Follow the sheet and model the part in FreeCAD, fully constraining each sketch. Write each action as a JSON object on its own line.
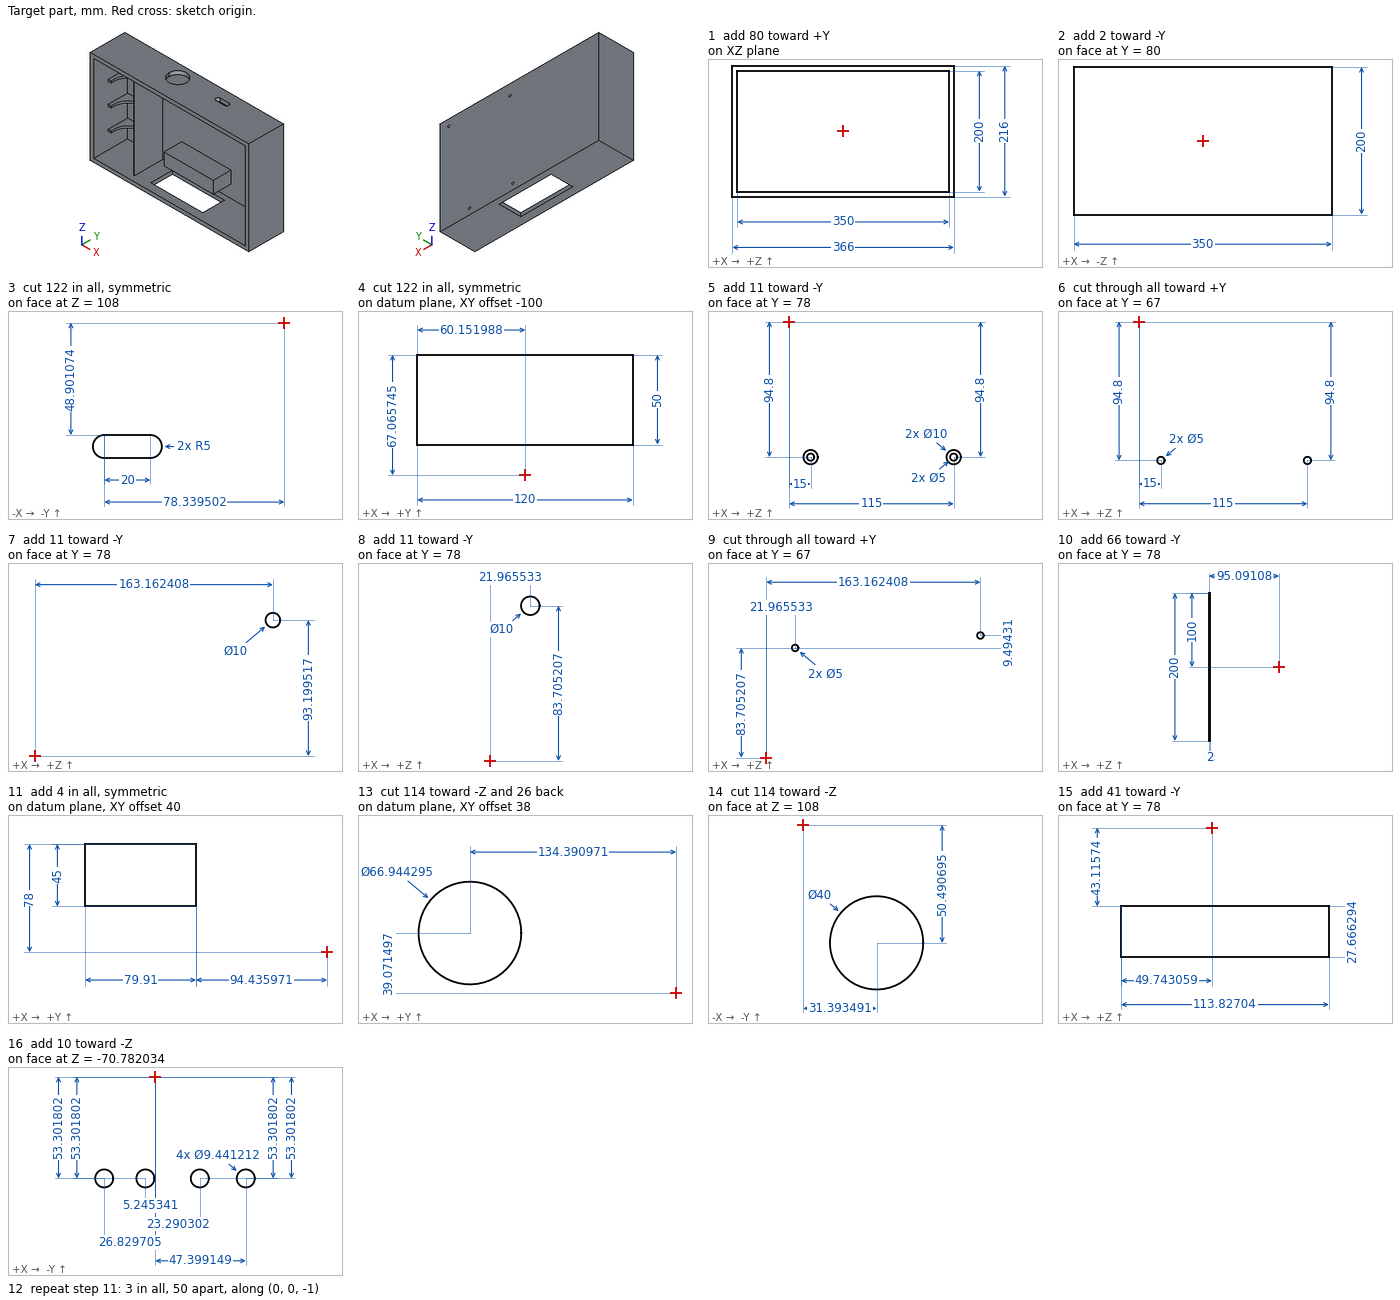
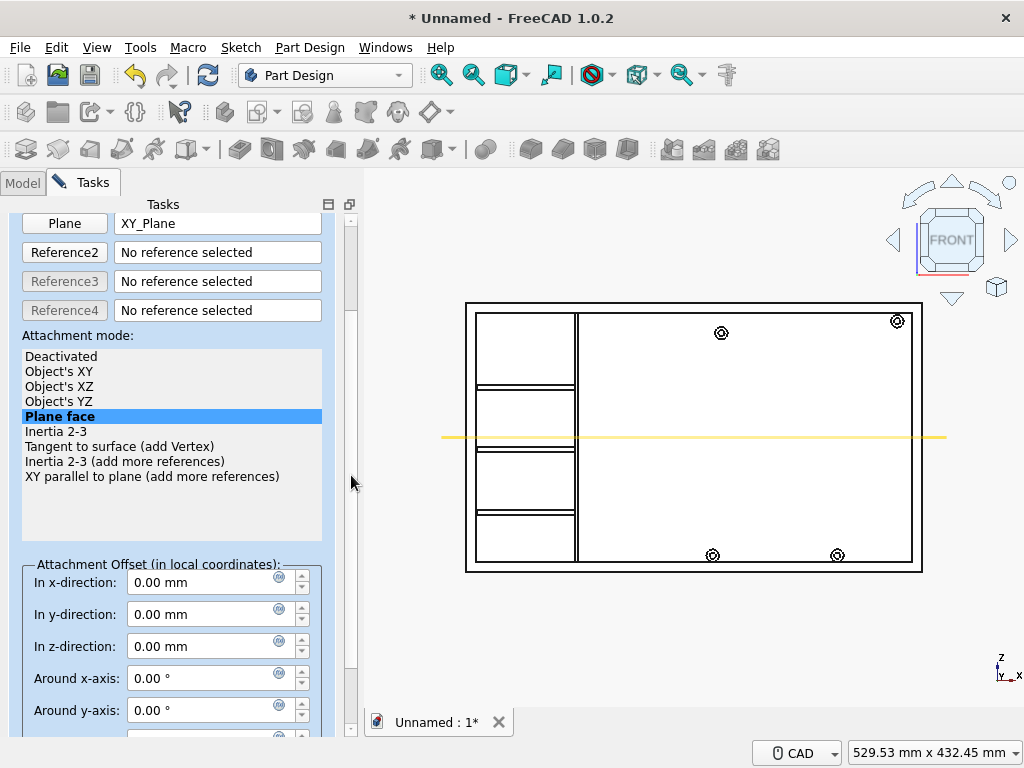
{"action": "triple_click", "coordinate": [210, 646]}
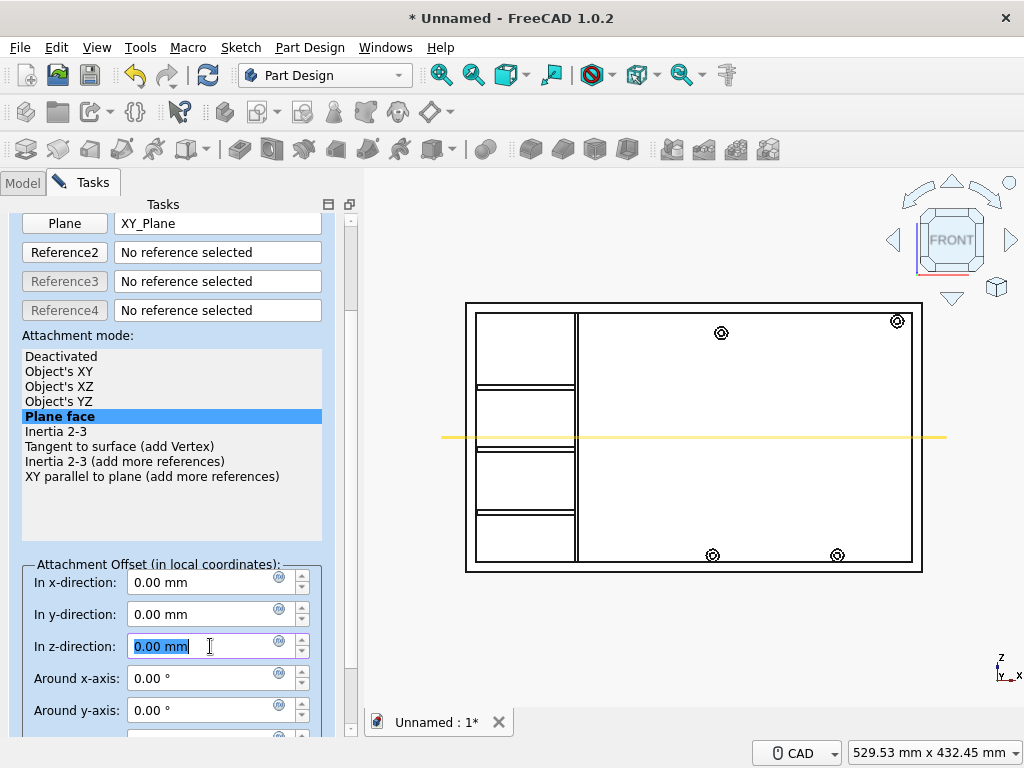
{"action": "type", "text": "38"}
{"action": "key", "text": "Tab"}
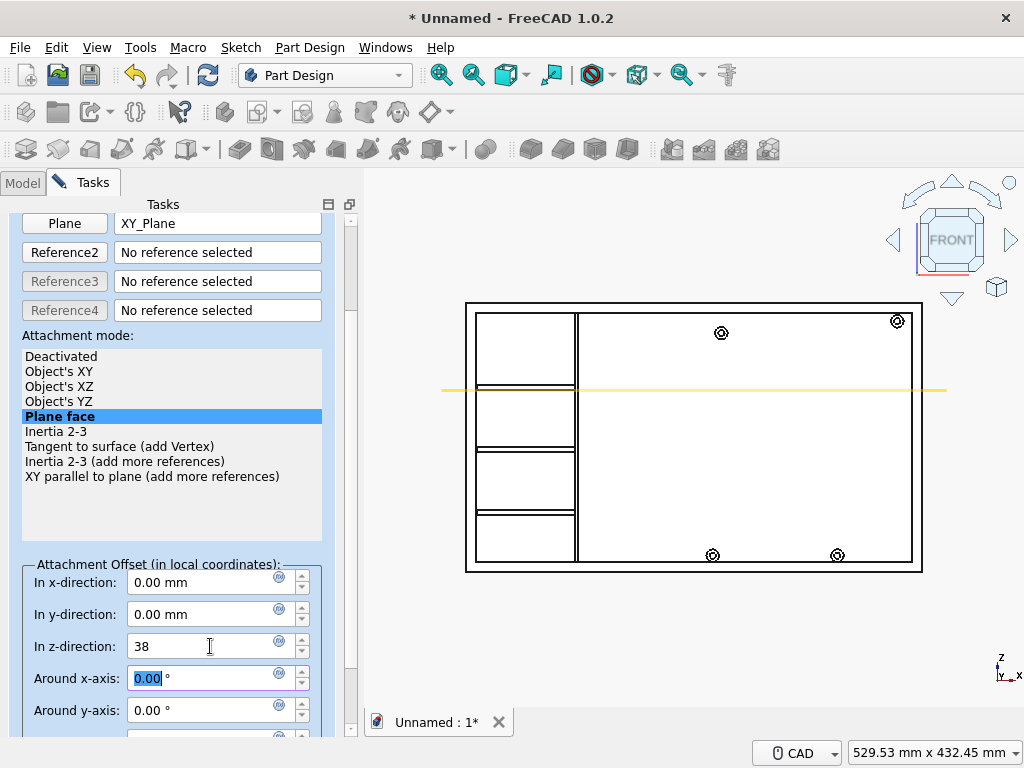
{"action": "scroll", "coordinate": [351, 475], "scroll_direction": "up", "scroll_amount": 3}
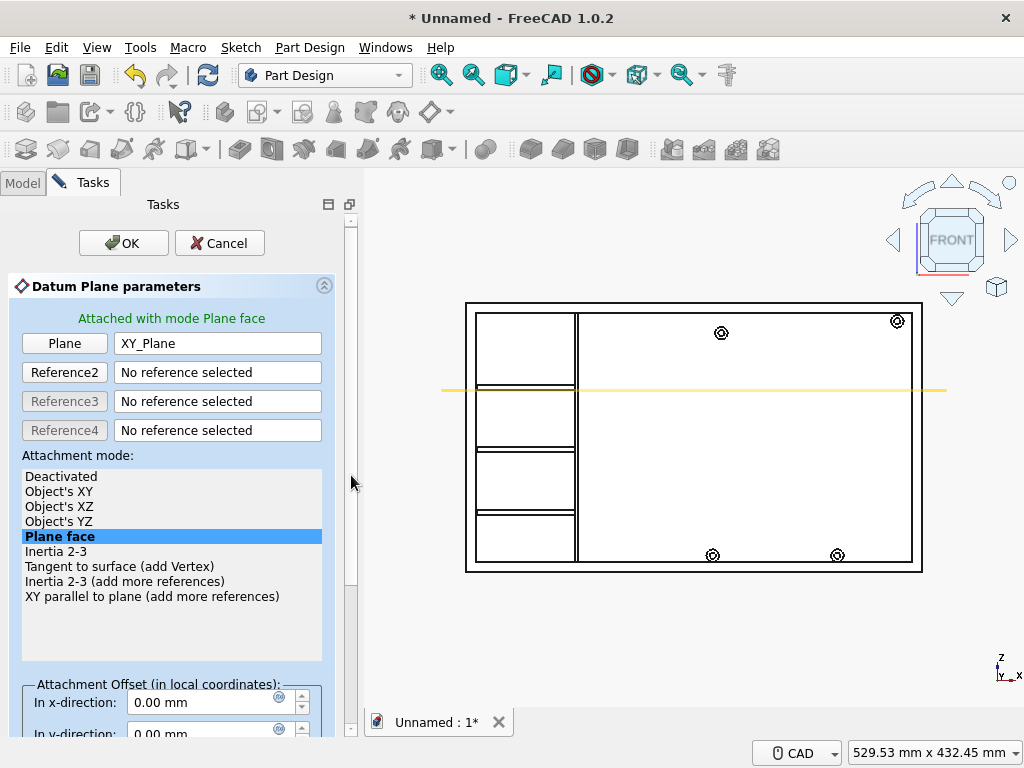
{"action": "left_click", "coordinate": [124, 243]}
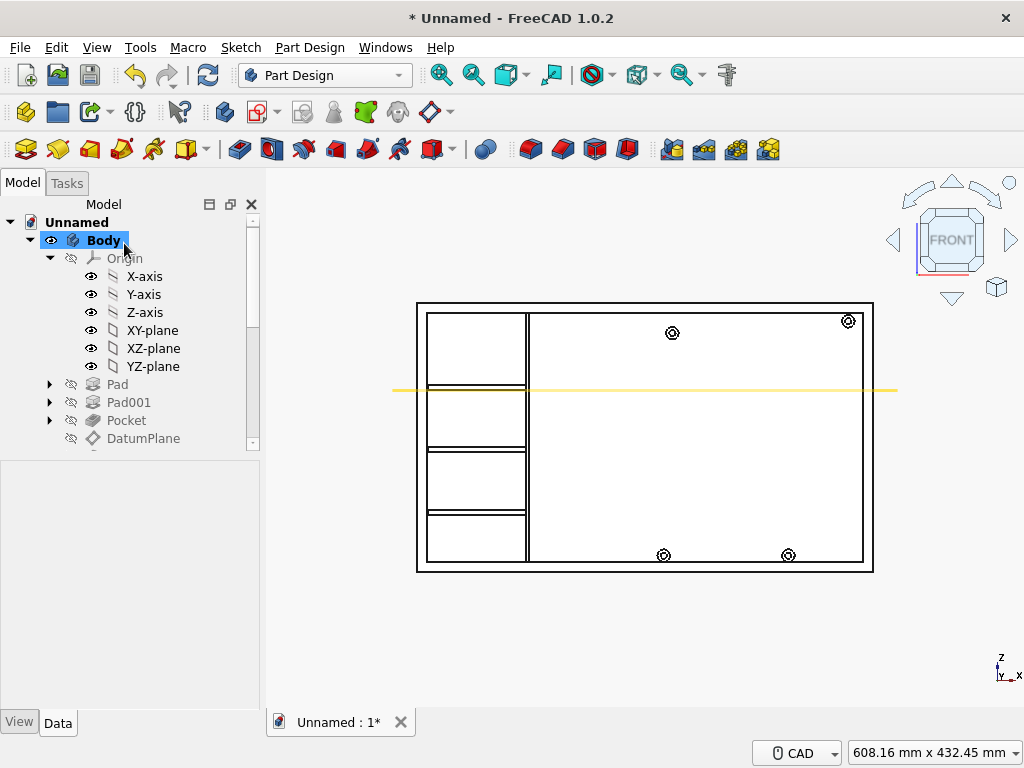
{"action": "scroll", "coordinate": [100, 326], "scroll_direction": "down", "scroll_amount": 3}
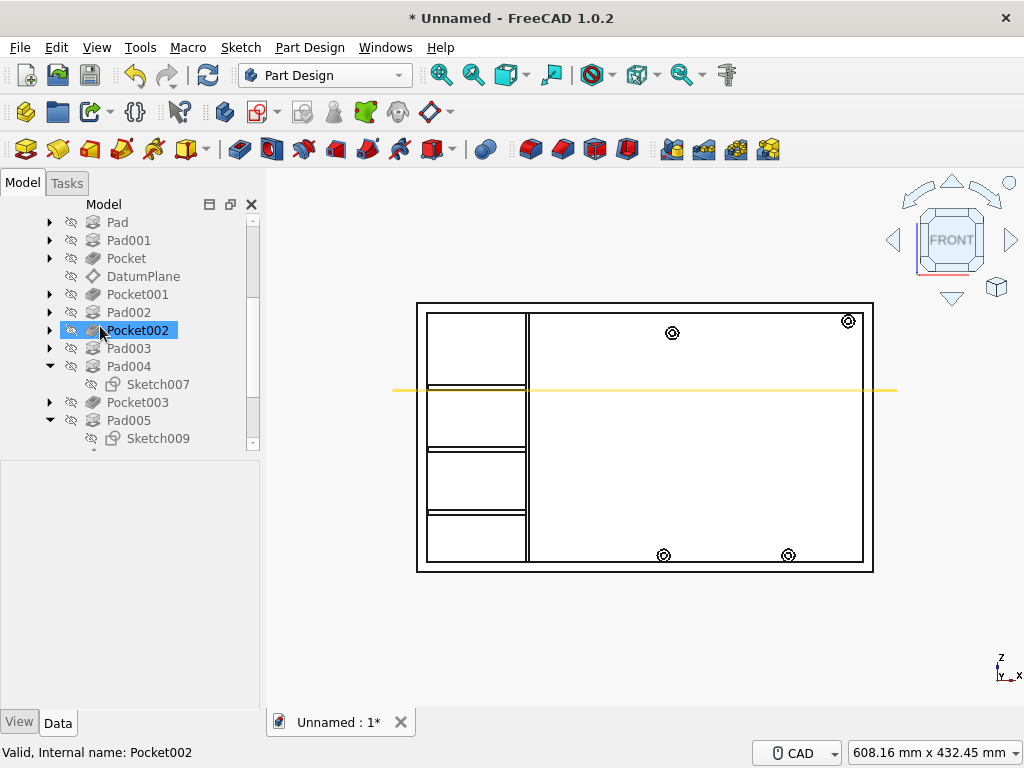
{"action": "scroll", "coordinate": [140, 326], "scroll_direction": "up", "scroll_amount": 15}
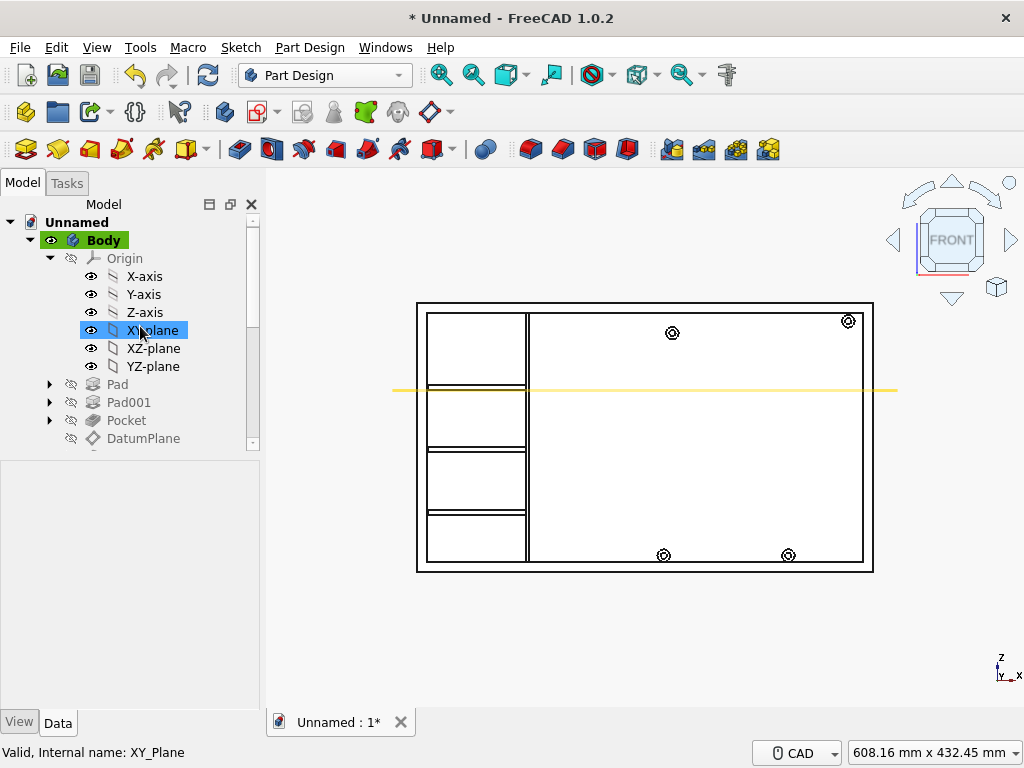
{"action": "scroll", "coordinate": [100, 326], "scroll_direction": "down", "scroll_amount": 6}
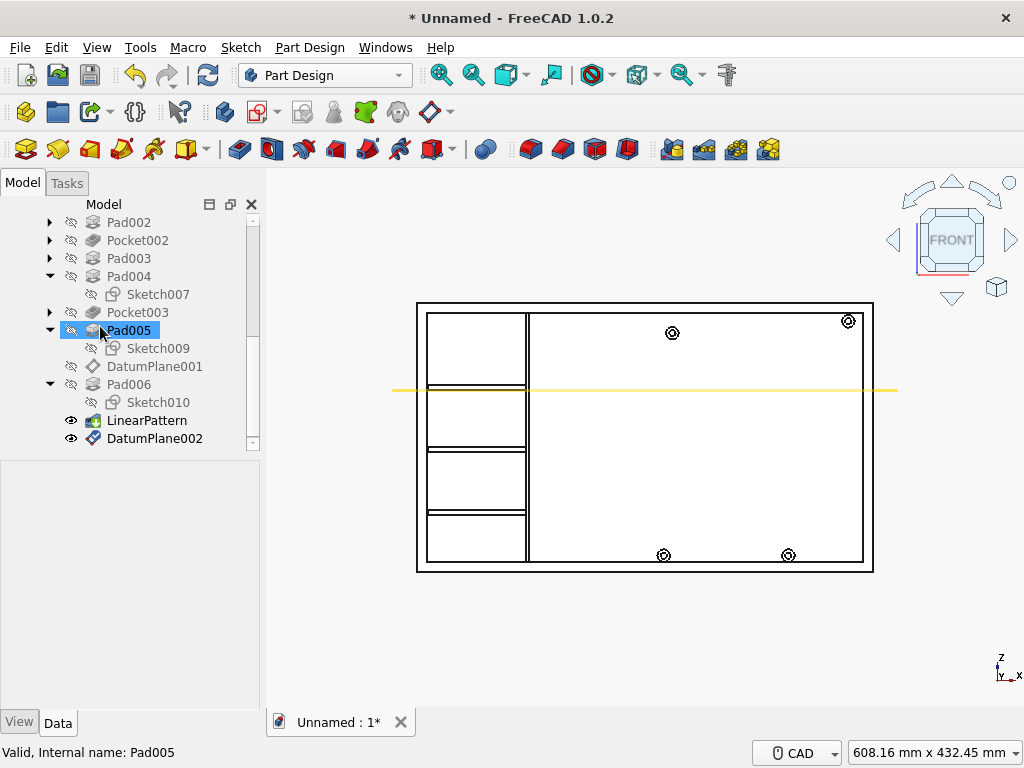
{"action": "left_click", "coordinate": [116, 438]}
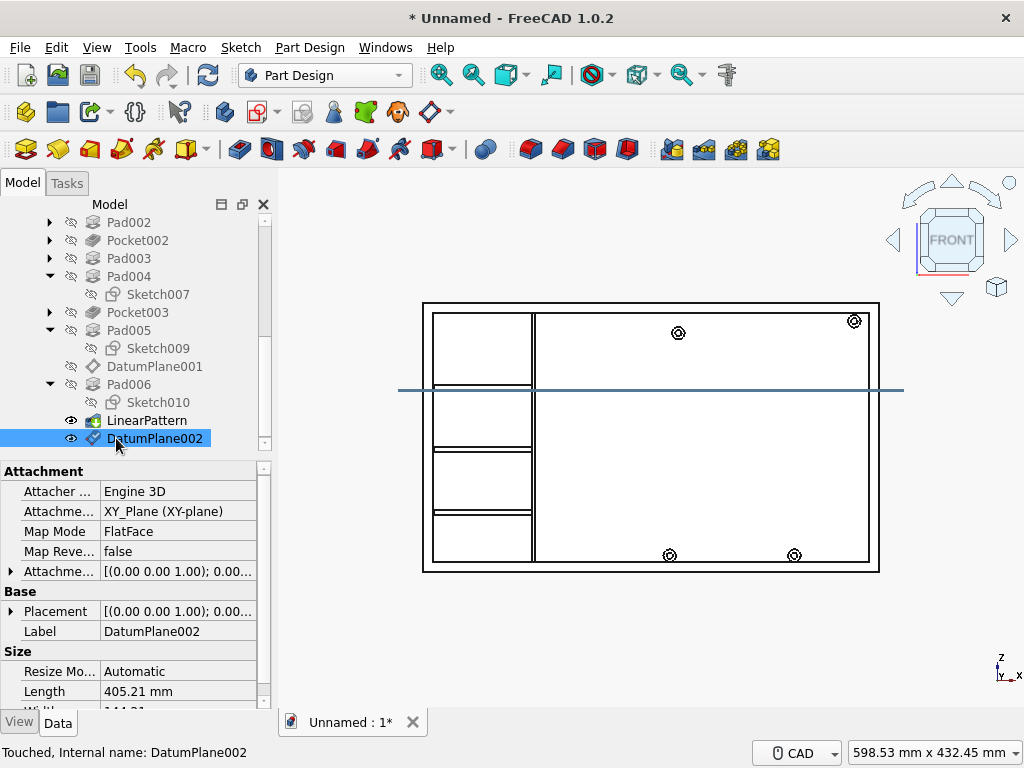
{"action": "left_click", "coordinate": [258, 112]}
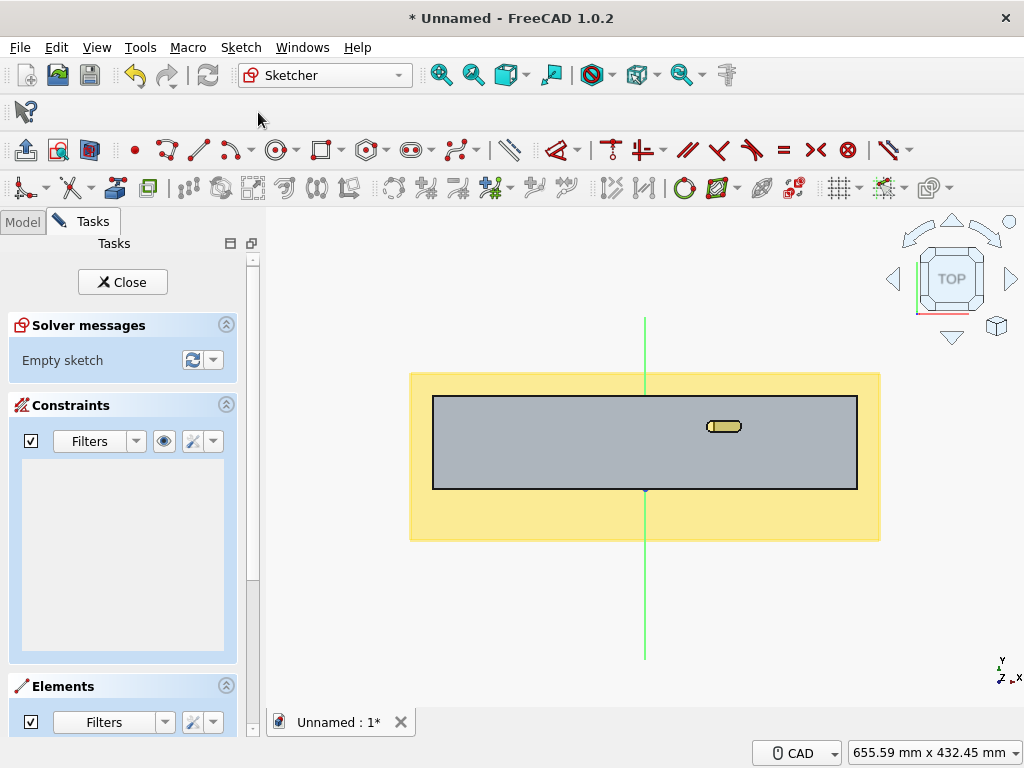
{"action": "left_click", "coordinate": [90, 150]}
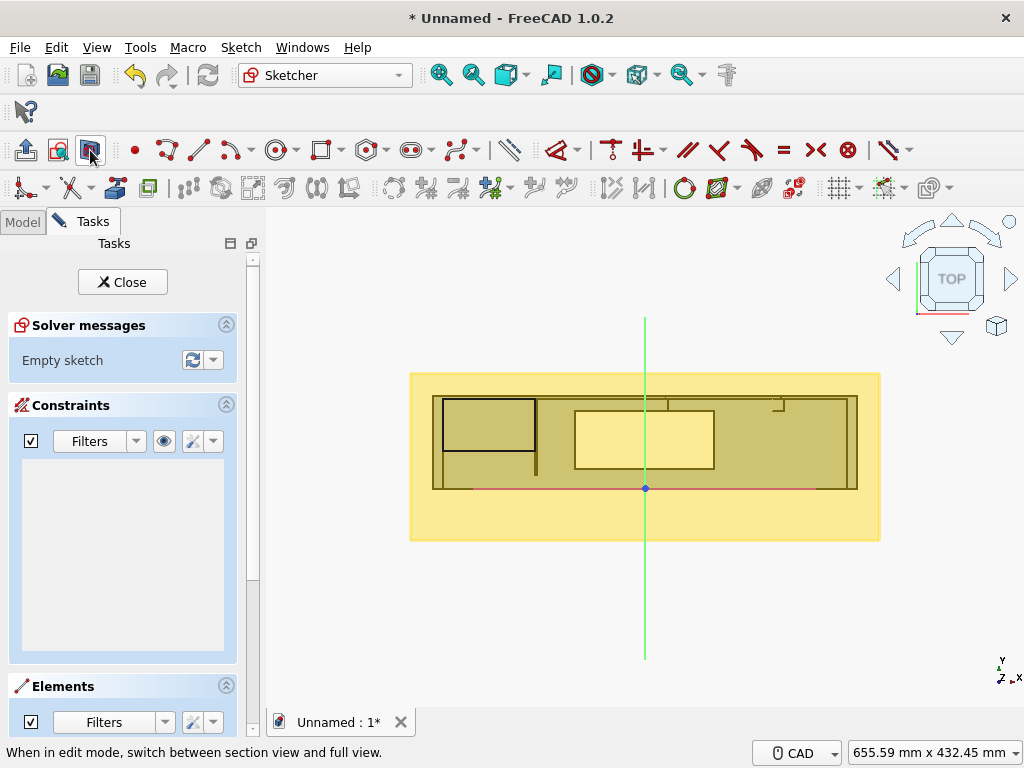
{"action": "scroll", "coordinate": [461, 439], "scroll_direction": "up", "scroll_amount": 7}